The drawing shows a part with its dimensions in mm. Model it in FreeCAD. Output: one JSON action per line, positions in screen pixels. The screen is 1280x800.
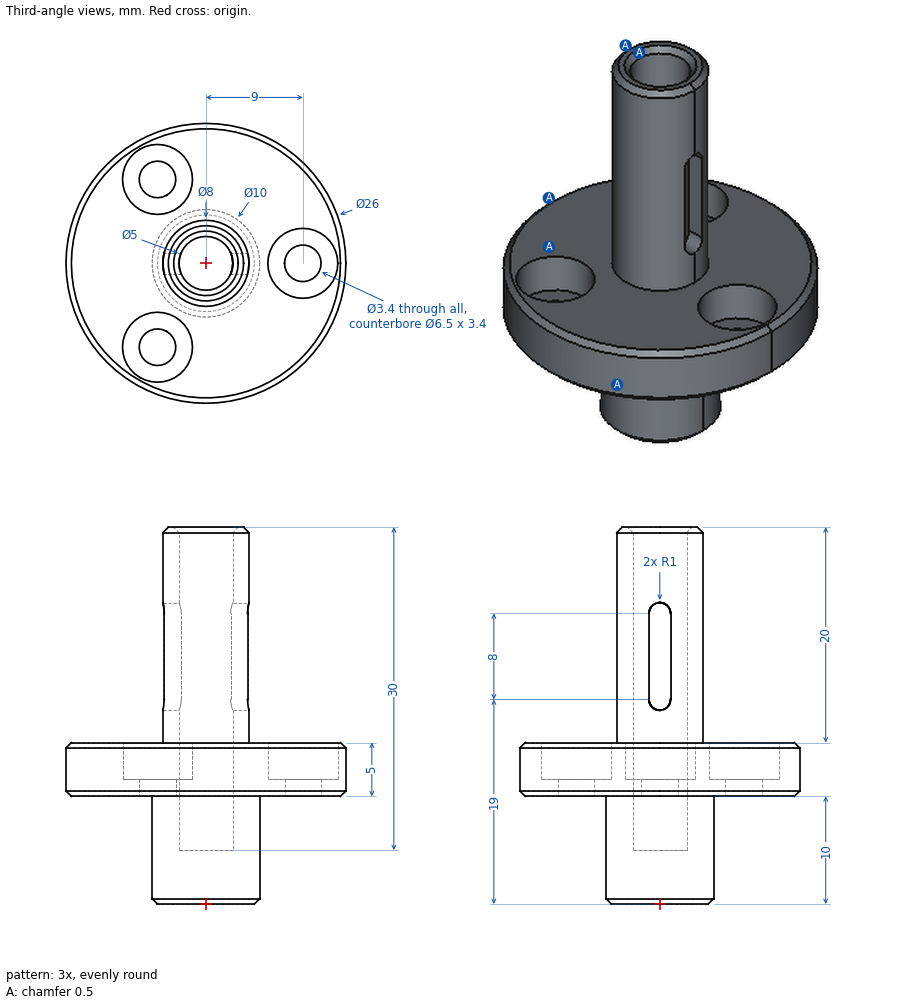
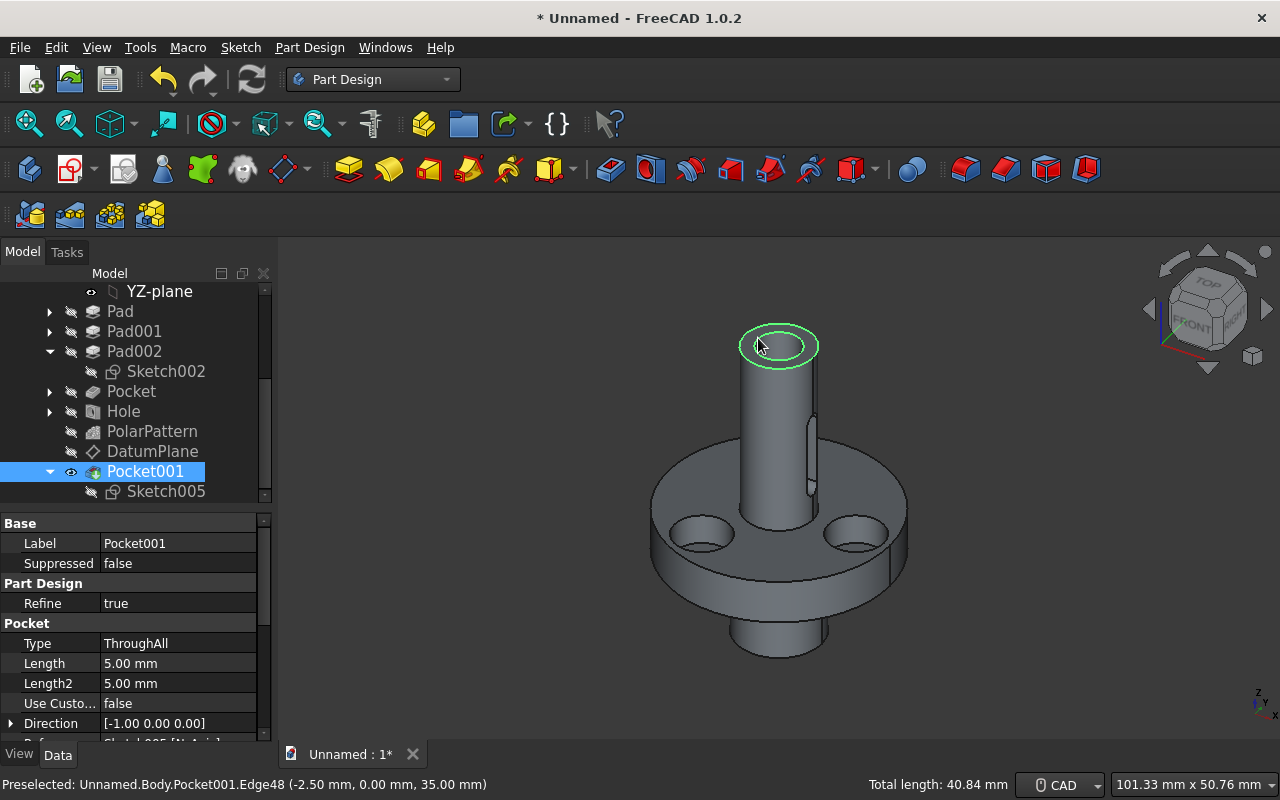
{"action": "left_click", "coordinate": [793, 656], "text": "ctrl"}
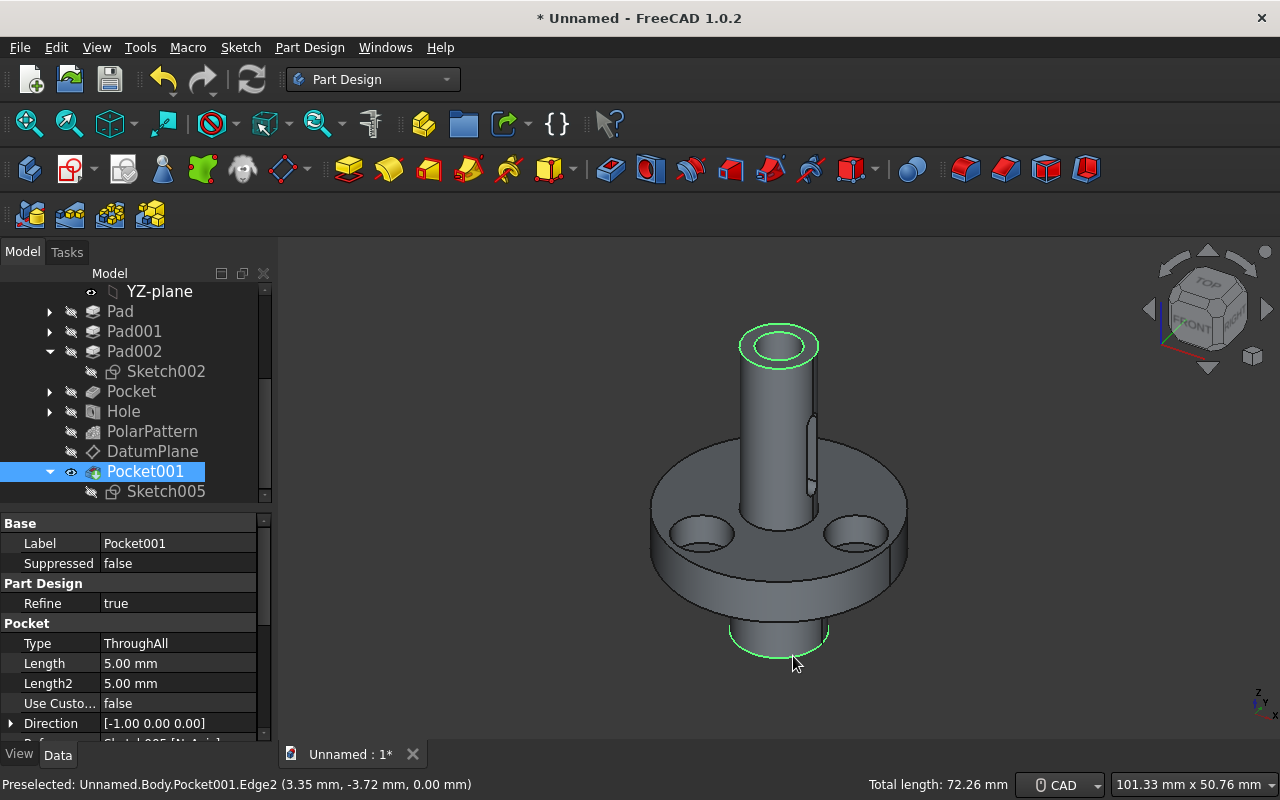
{"action": "left_click", "coordinate": [651, 515], "text": "ctrl"}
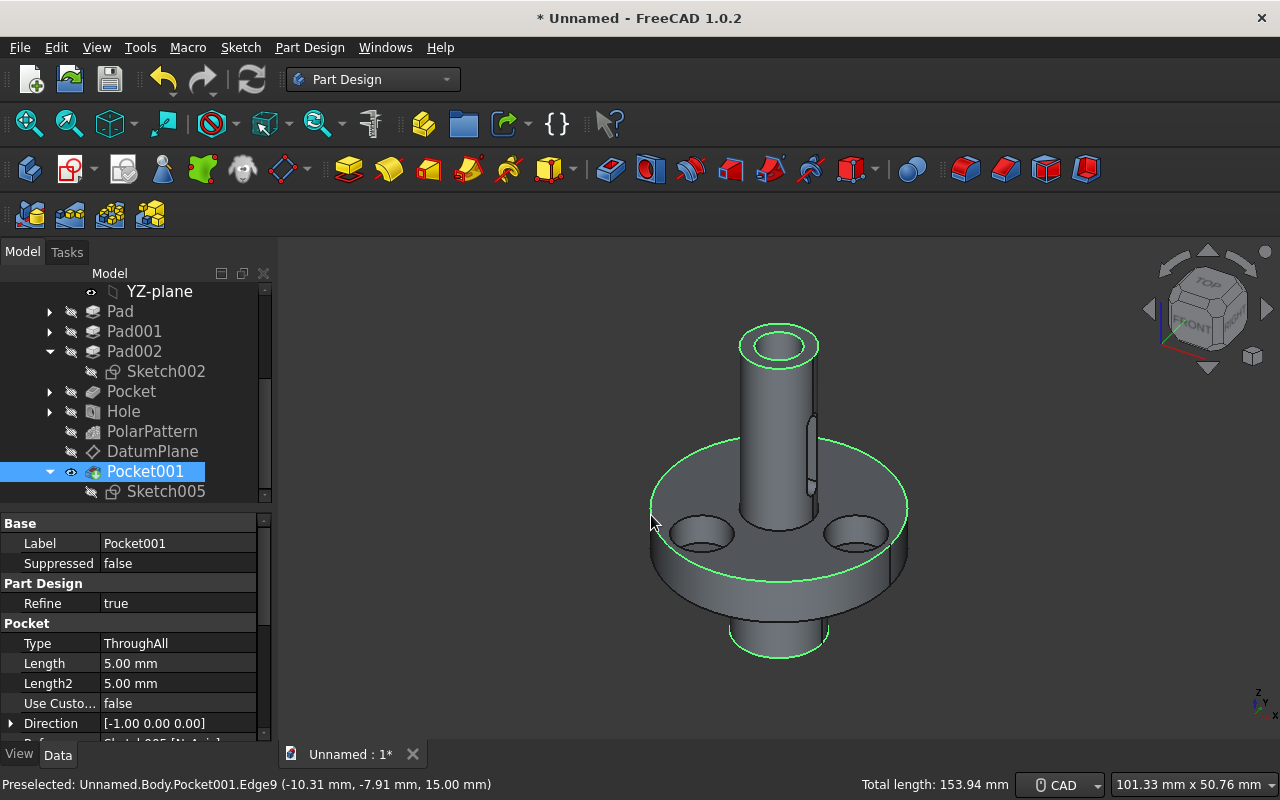
{"action": "key", "text": "0"}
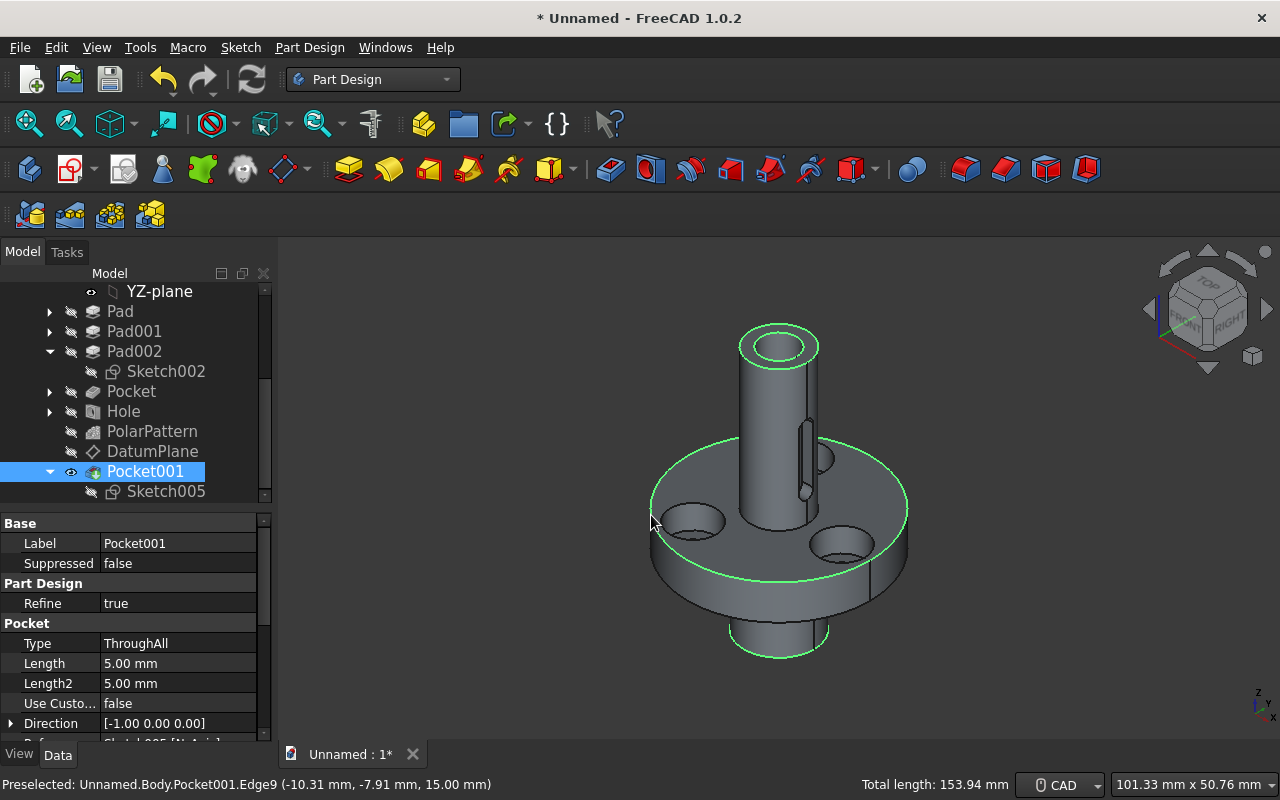
{"action": "key", "text": "2"}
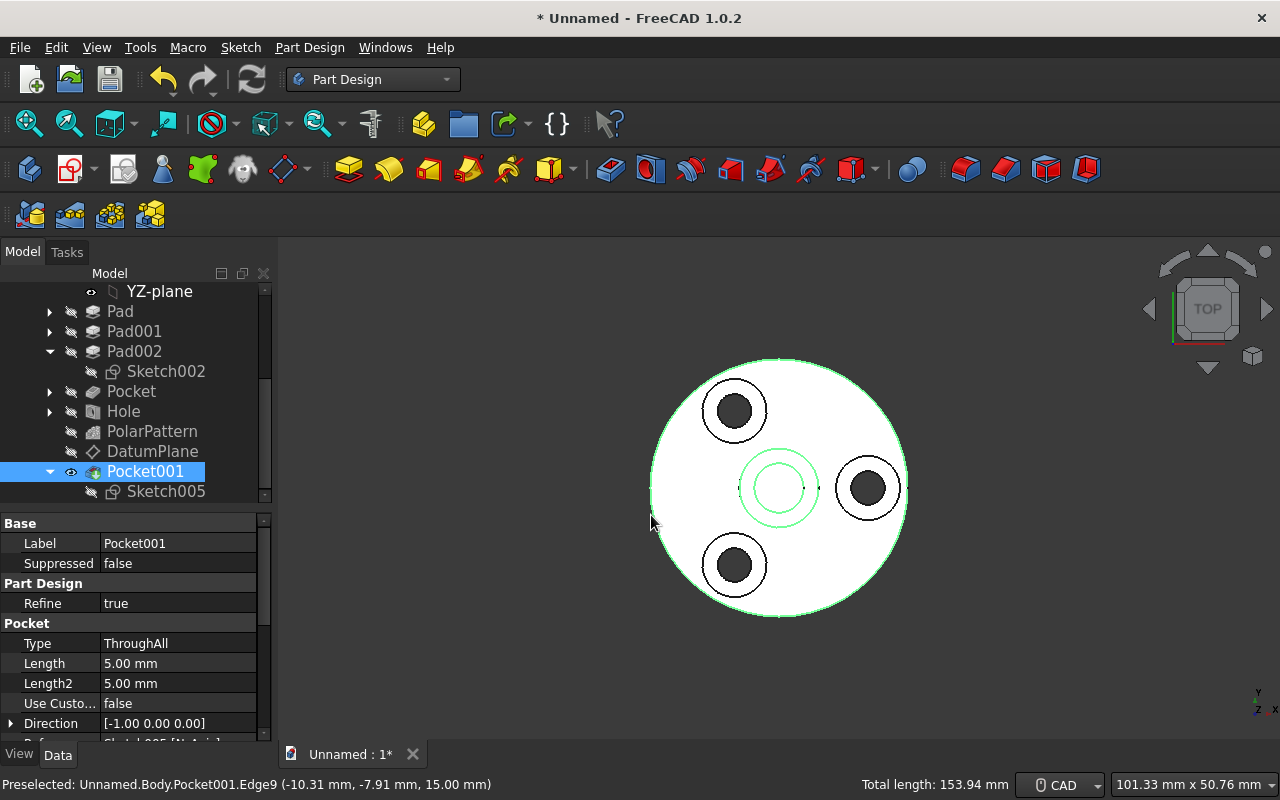
{"action": "key", "text": "1"}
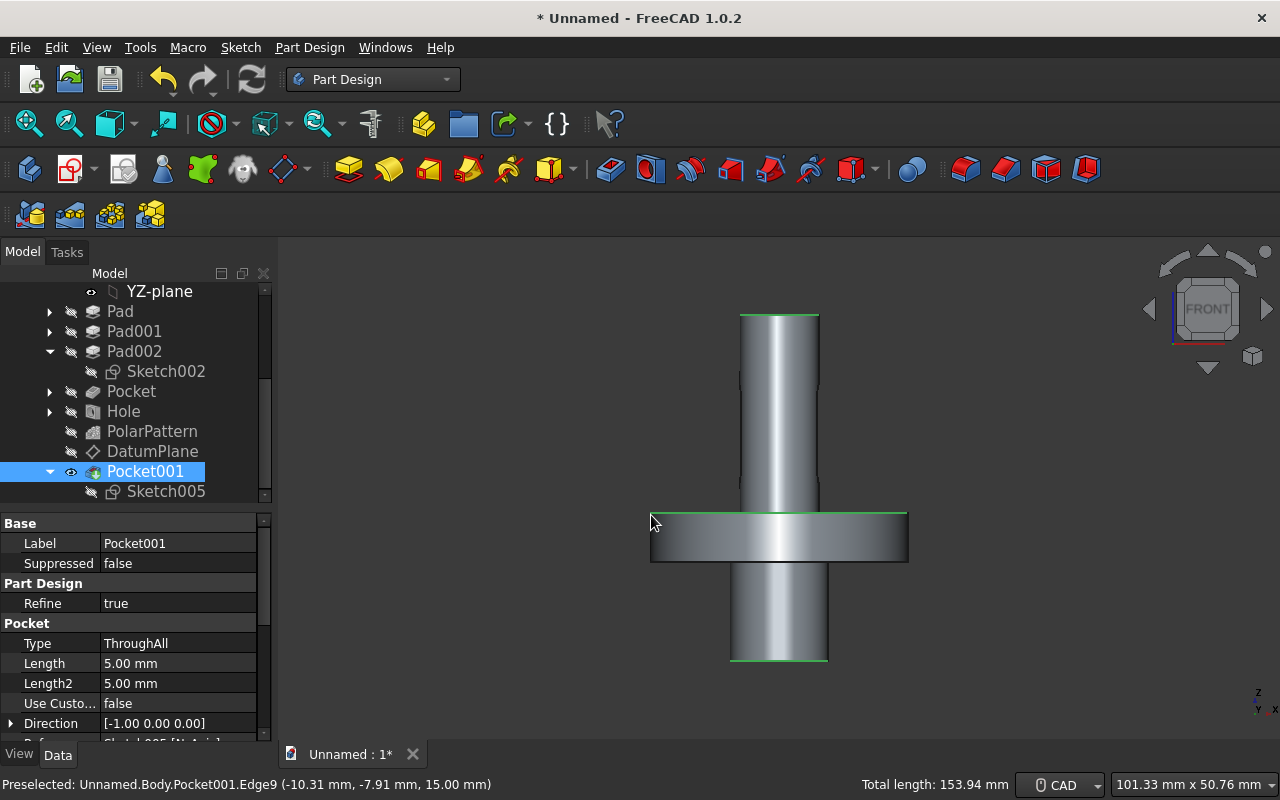
{"action": "left_click", "coordinate": [675, 561], "text": "ctrl"}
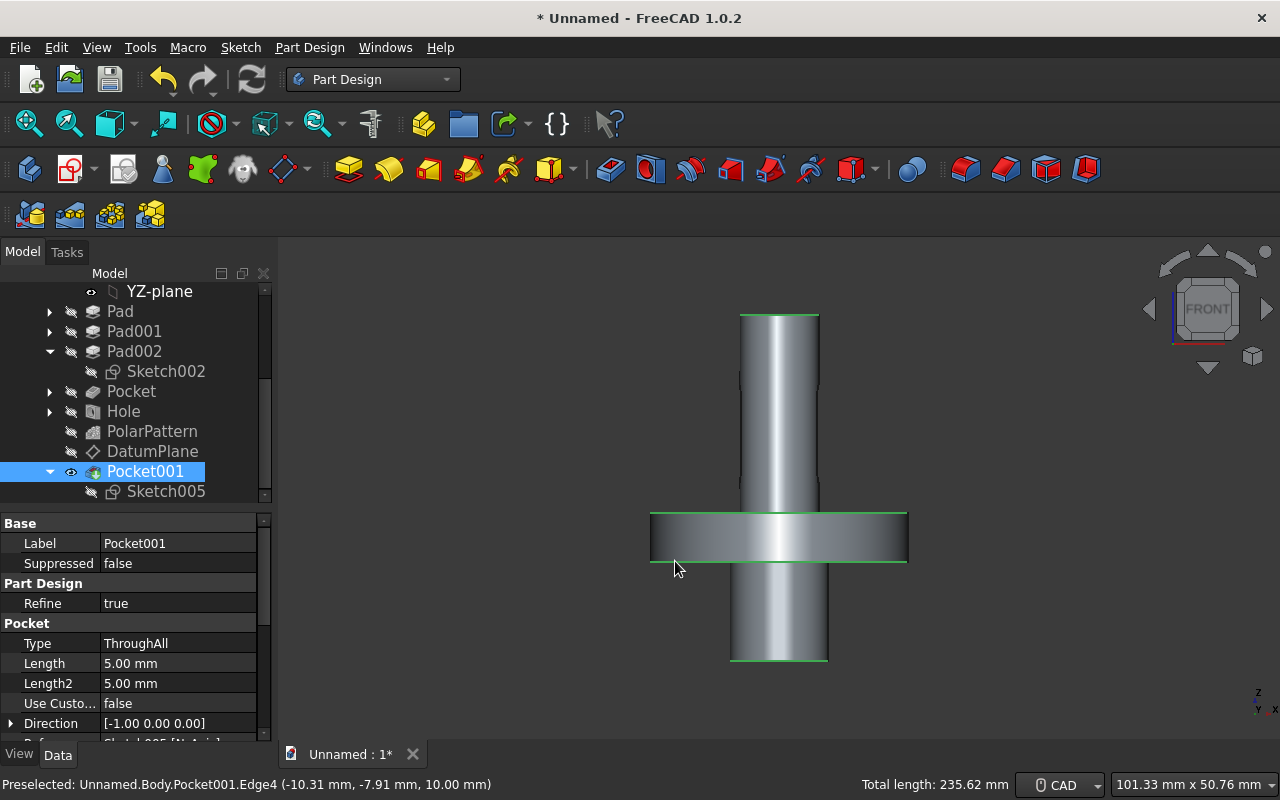
{"action": "left_click", "coordinate": [1006, 170]}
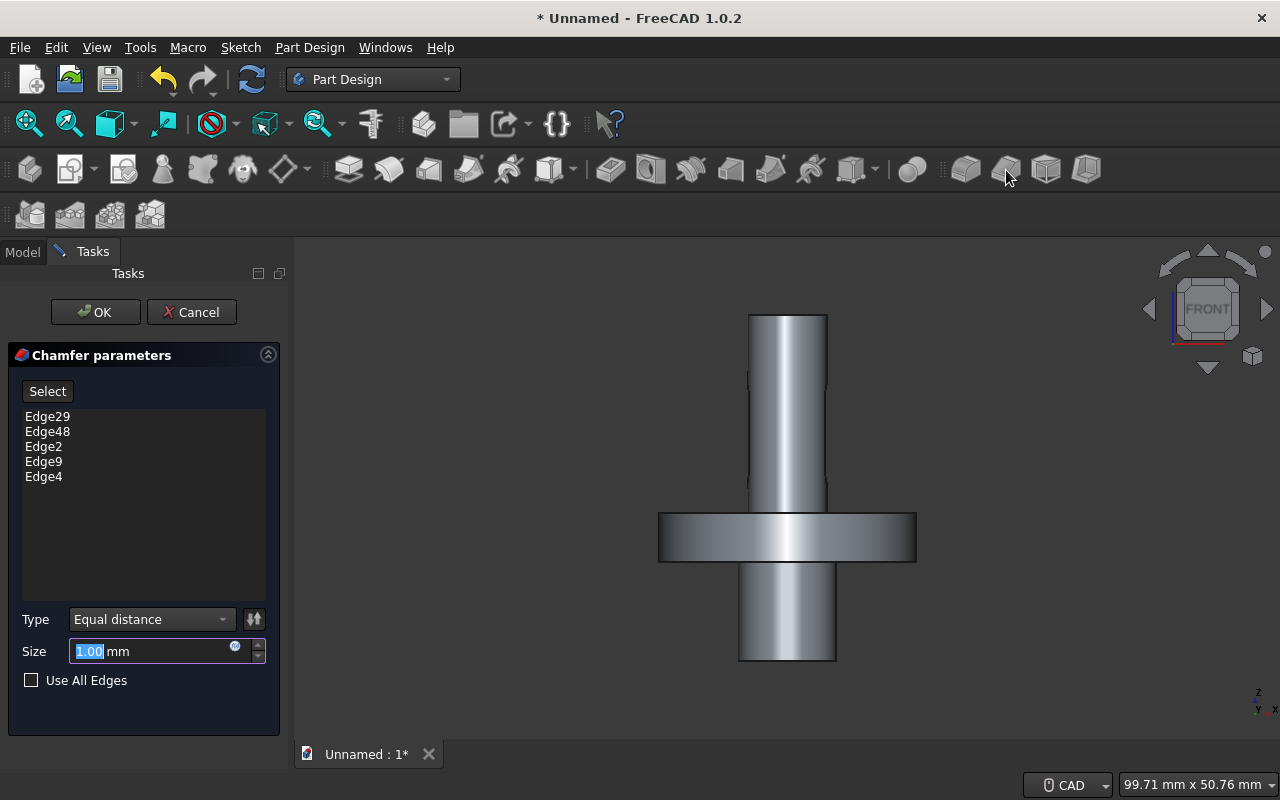
{"action": "type", "text": "0.5"}
{"action": "key", "text": "Tab"}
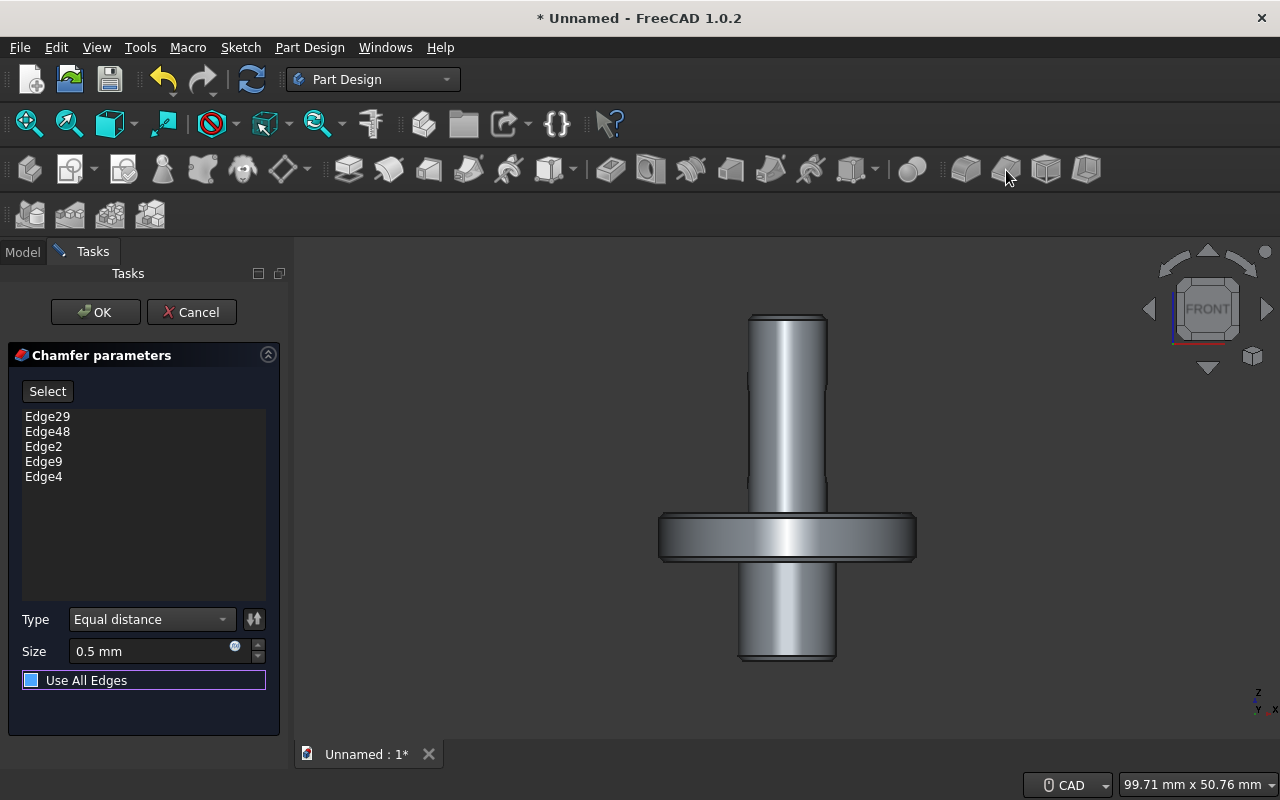
{"action": "left_click", "coordinate": [96, 312]}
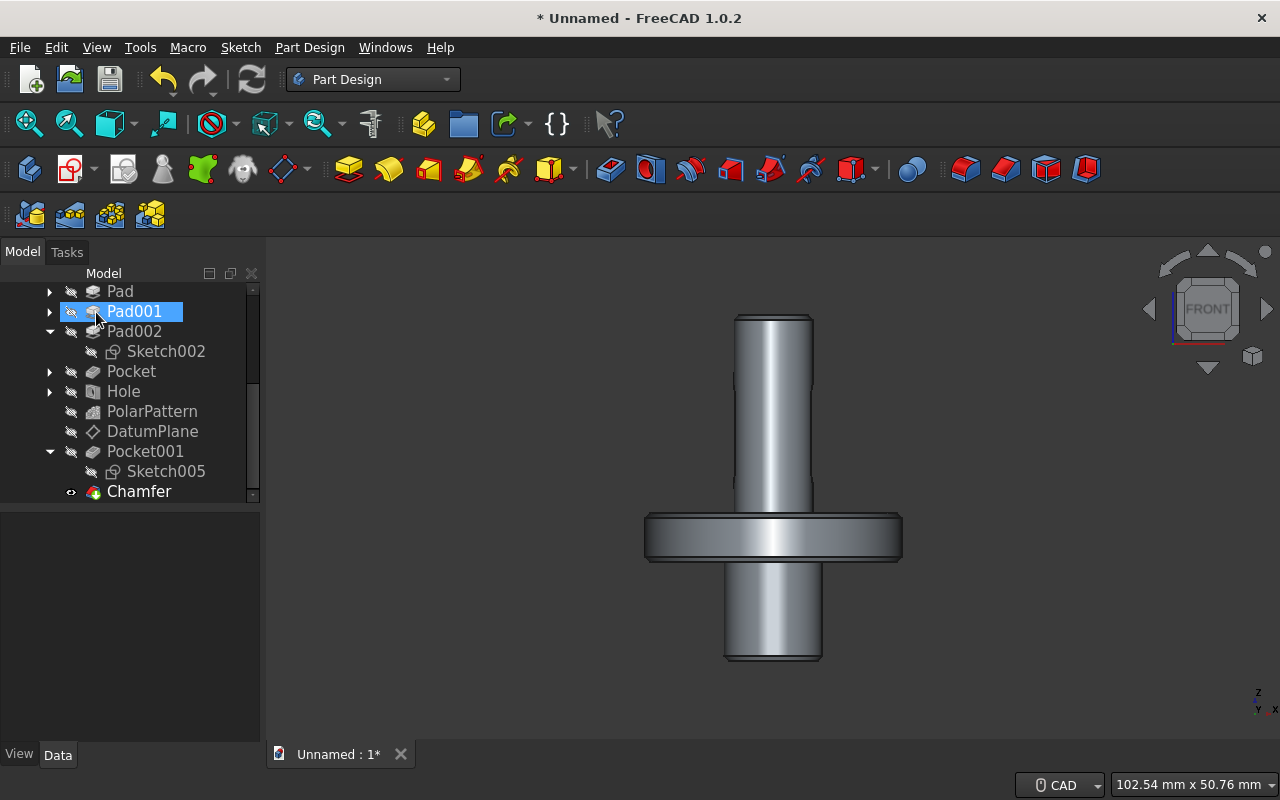
{"action": "key", "text": "0"}